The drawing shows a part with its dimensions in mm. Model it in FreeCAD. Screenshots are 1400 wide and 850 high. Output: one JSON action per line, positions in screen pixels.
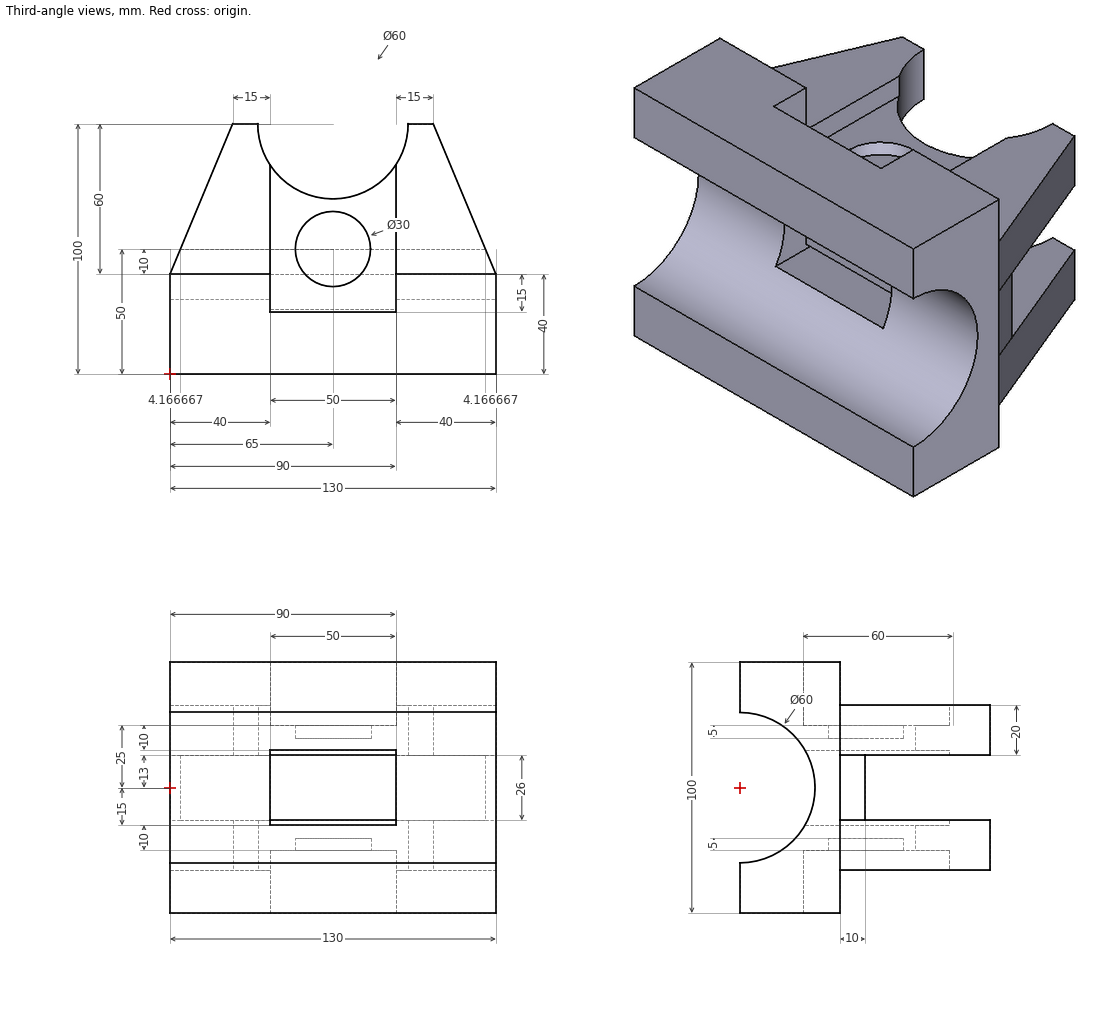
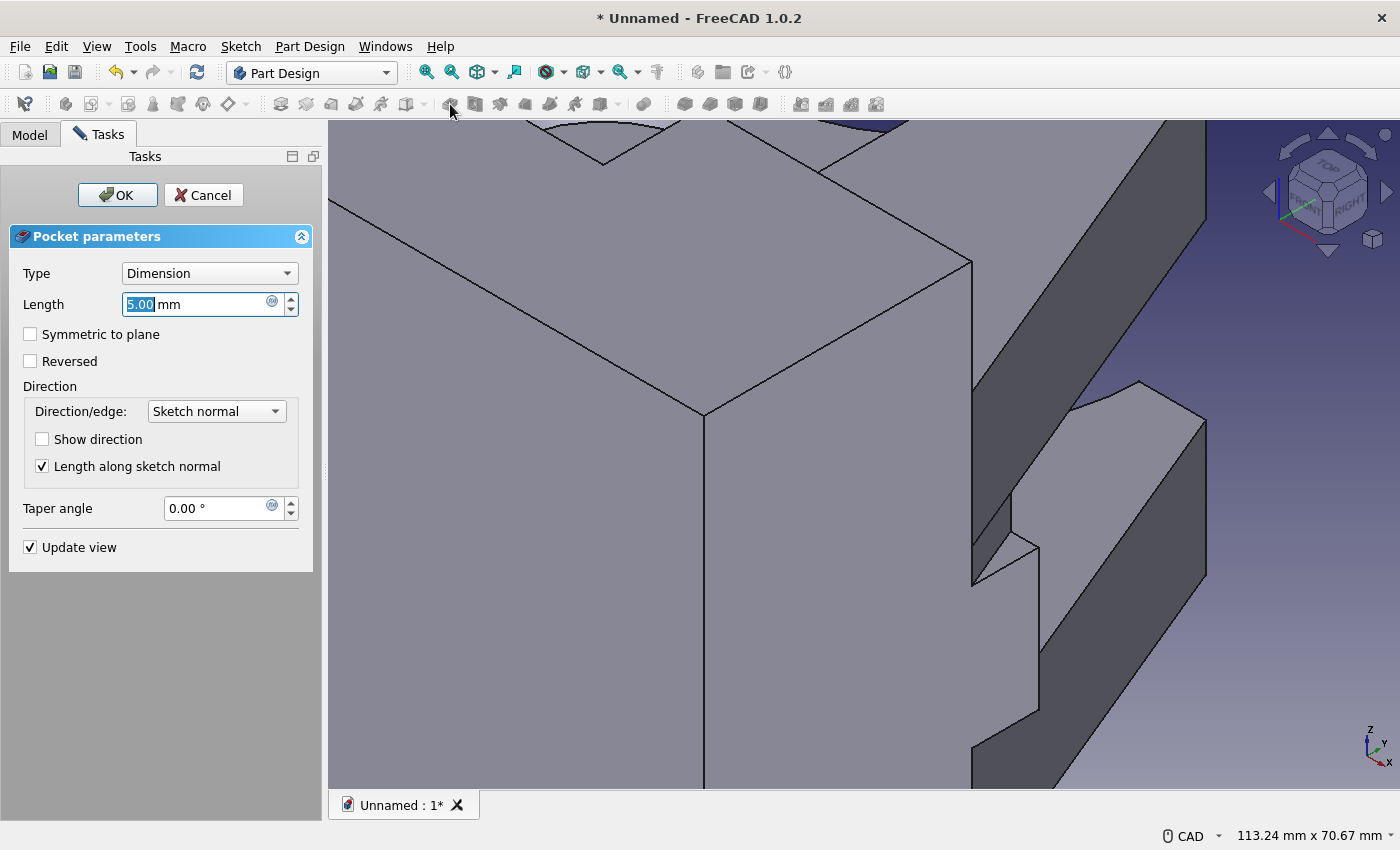
{"action": "left_click", "coordinate": [210, 274]}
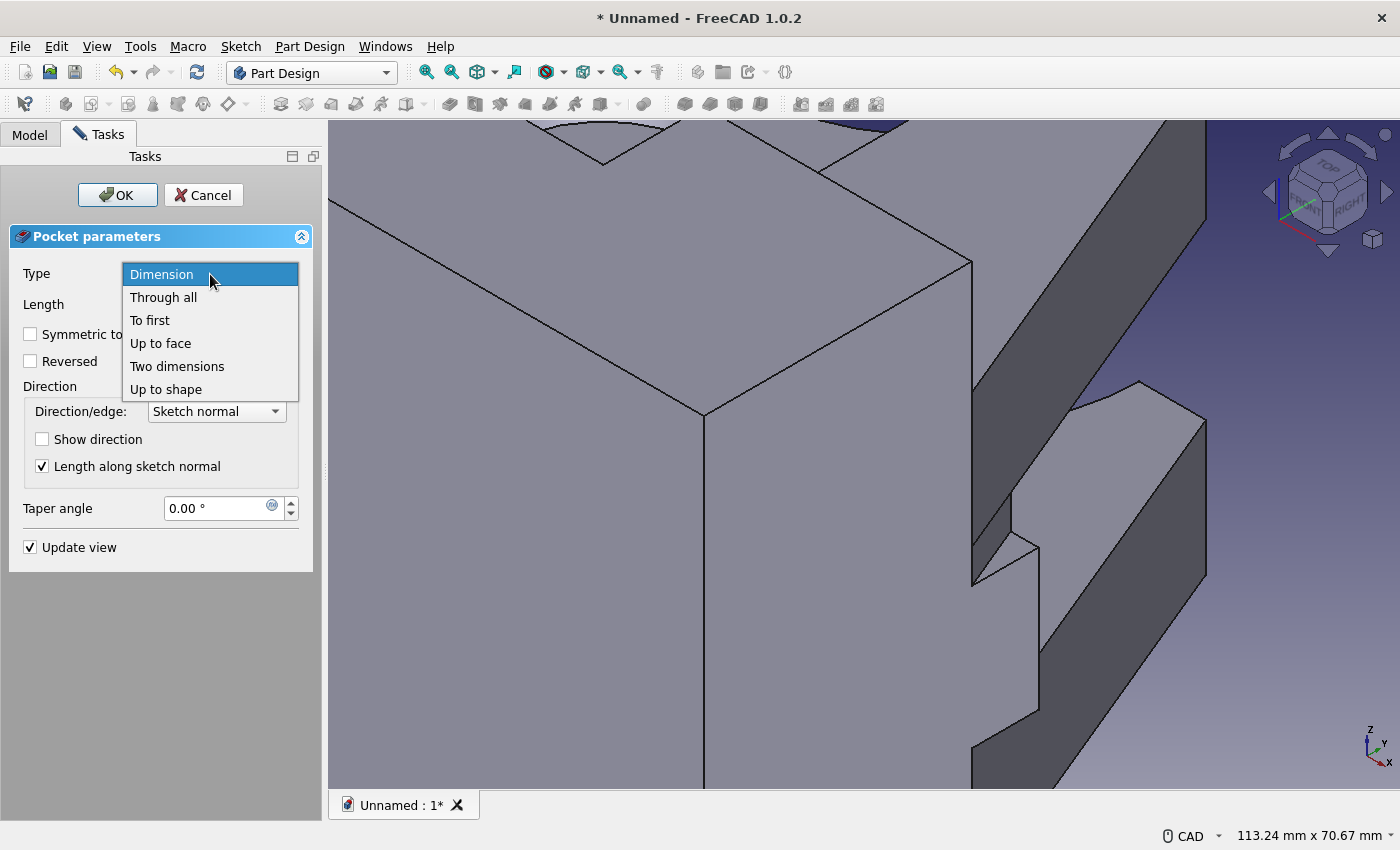
{"action": "left_click", "coordinate": [208, 298]}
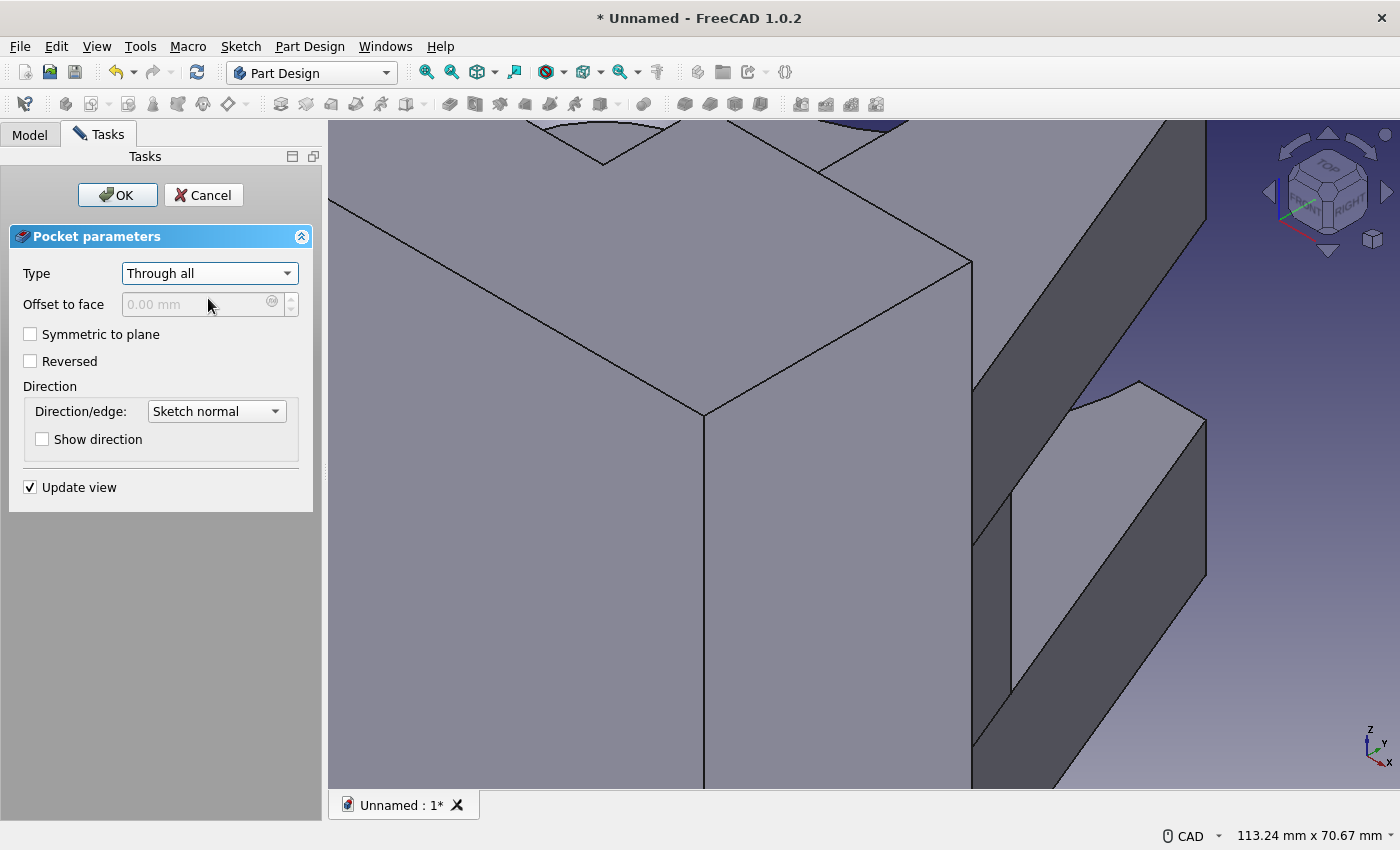
{"action": "left_click", "coordinate": [118, 195]}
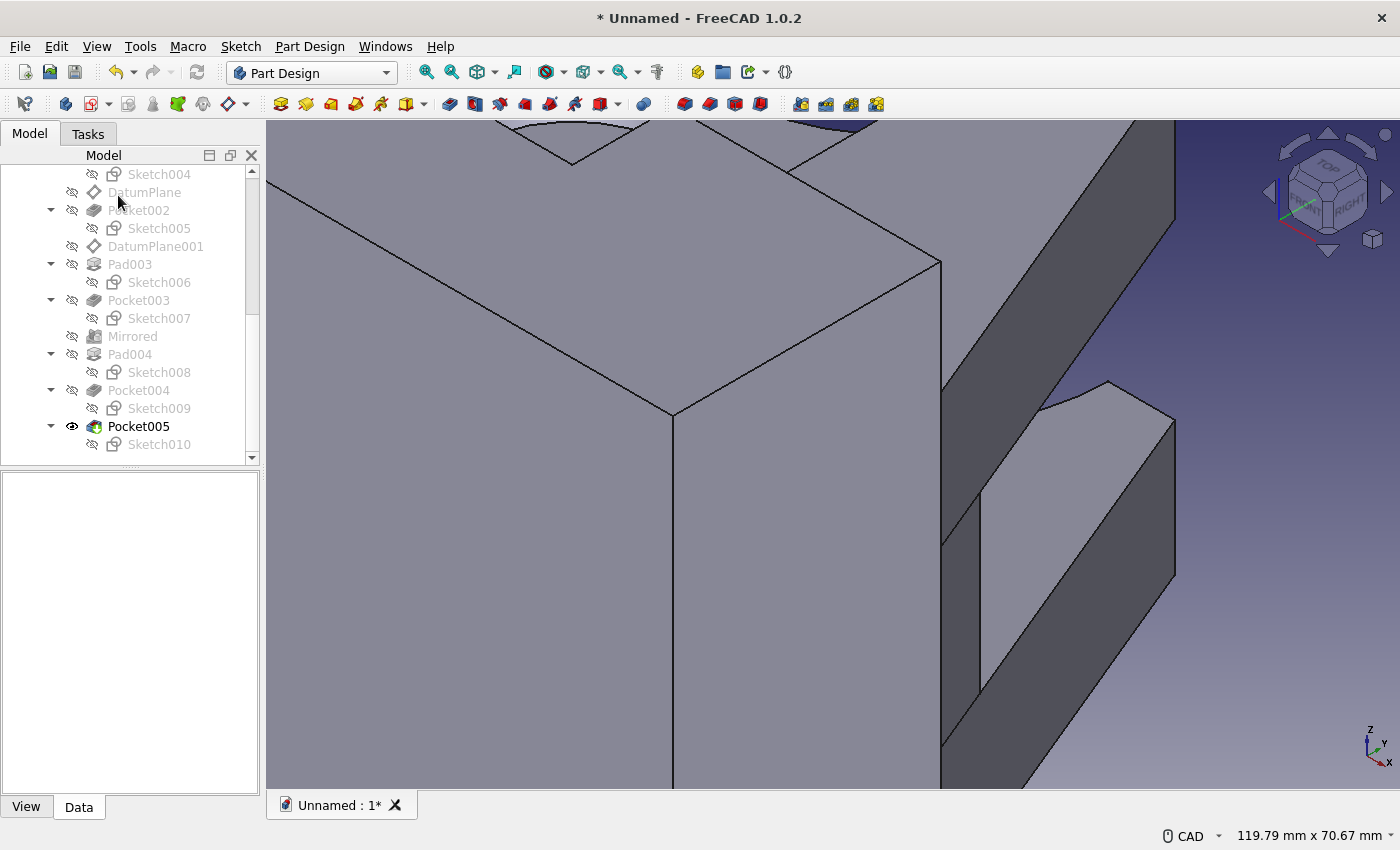
{"action": "left_click", "coordinate": [427, 72]}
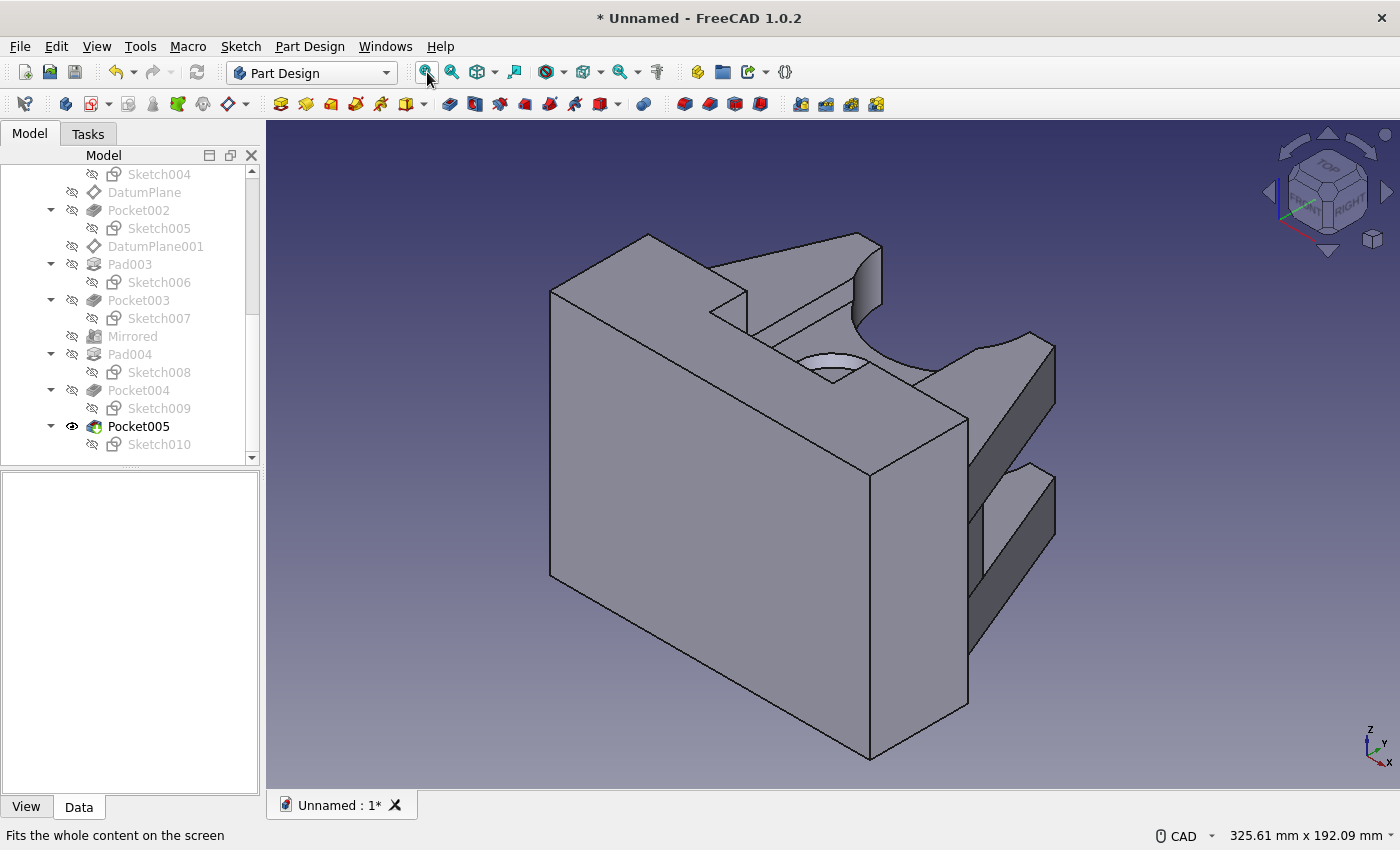
{"action": "left_click", "coordinate": [919, 507]}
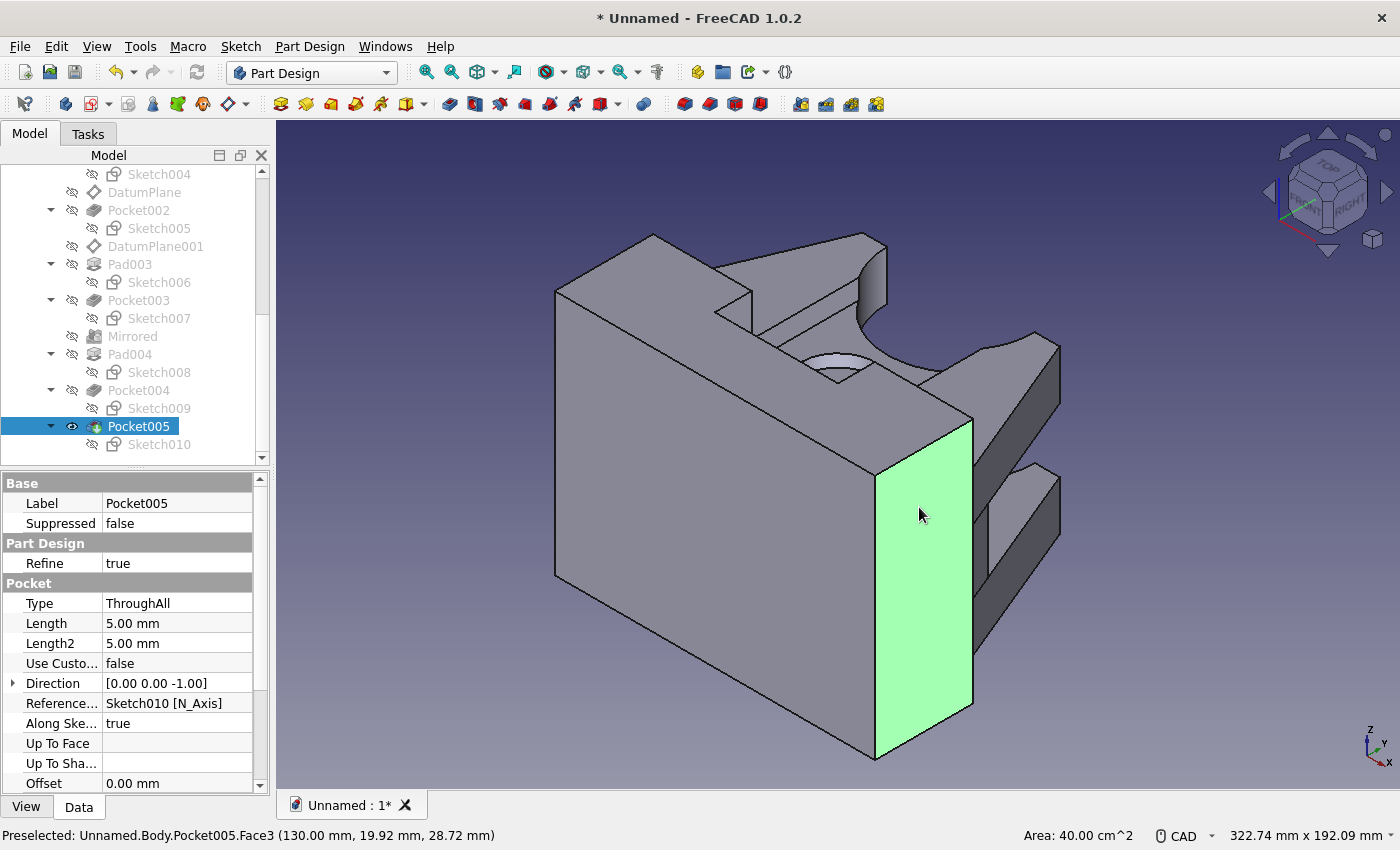
{"action": "left_click", "coordinate": [90, 104]}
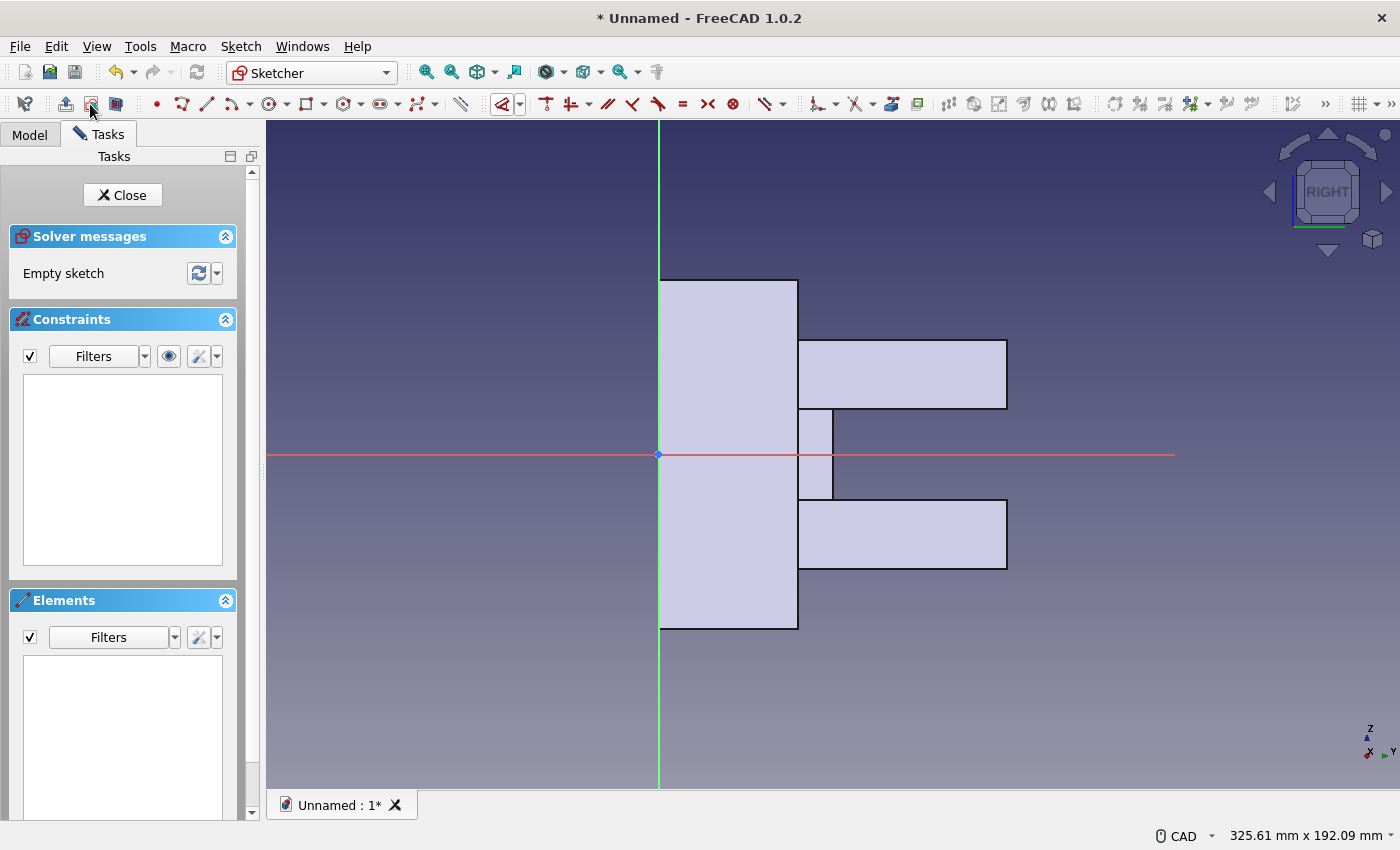
{"action": "scroll", "coordinate": [573, 455], "scroll_direction": "up", "scroll_amount": 4}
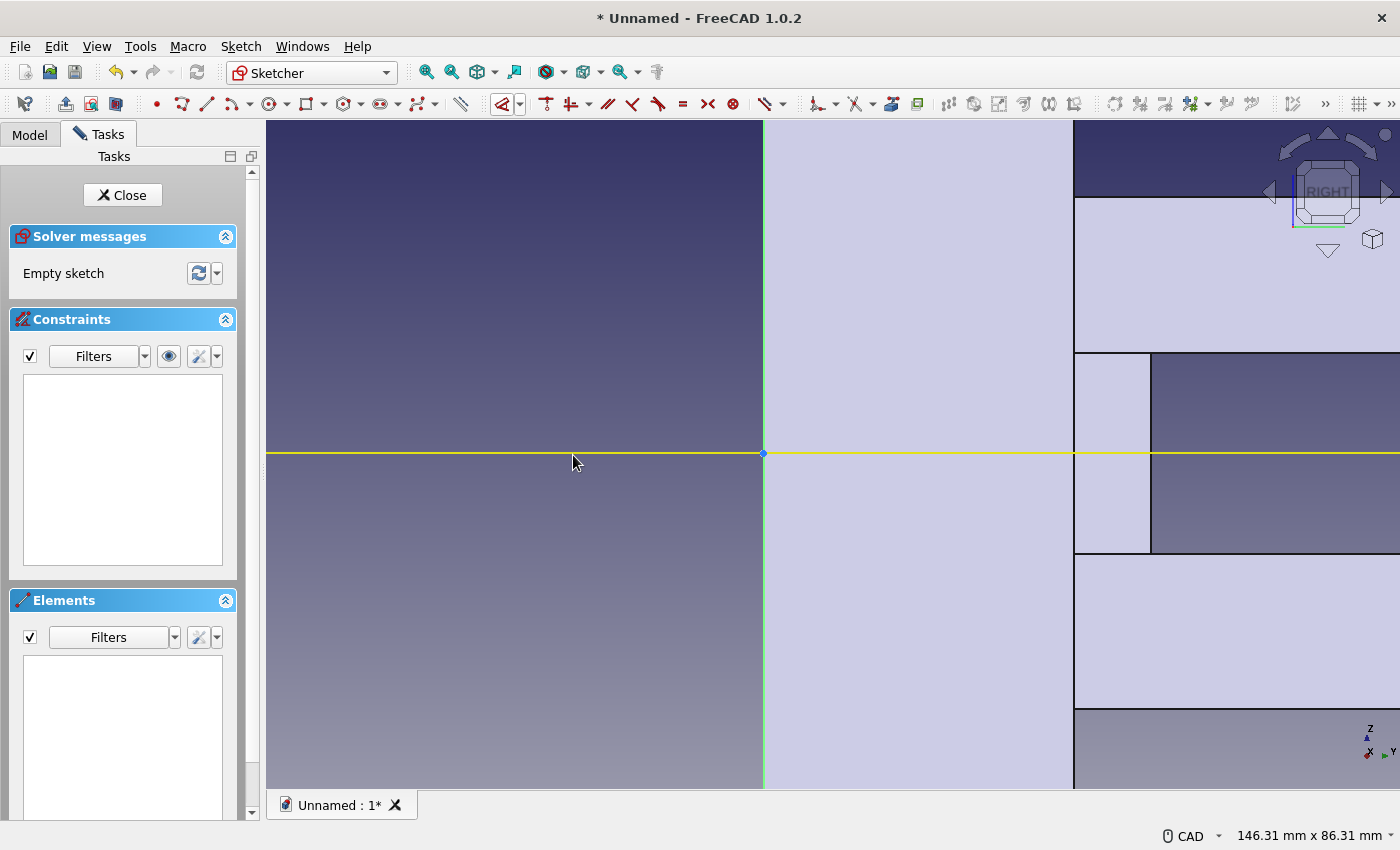
{"action": "left_click", "coordinate": [268, 104]}